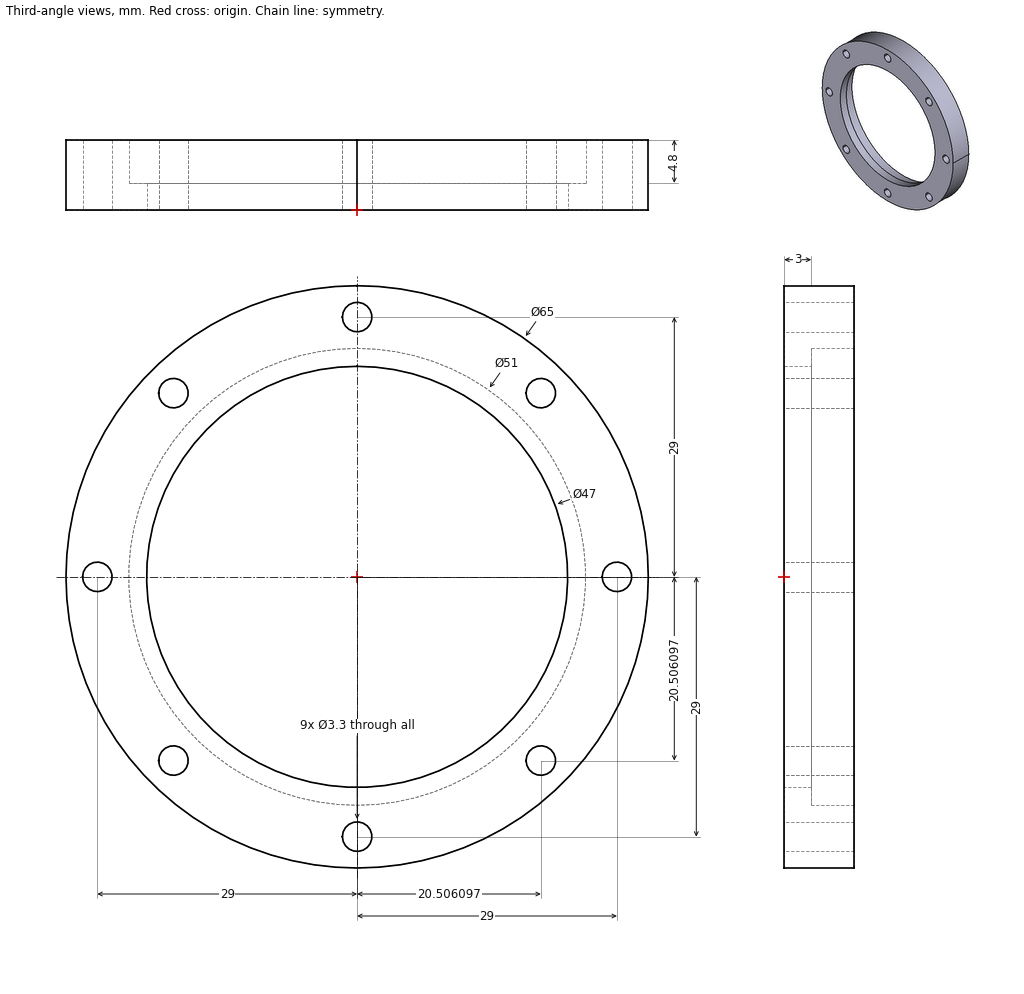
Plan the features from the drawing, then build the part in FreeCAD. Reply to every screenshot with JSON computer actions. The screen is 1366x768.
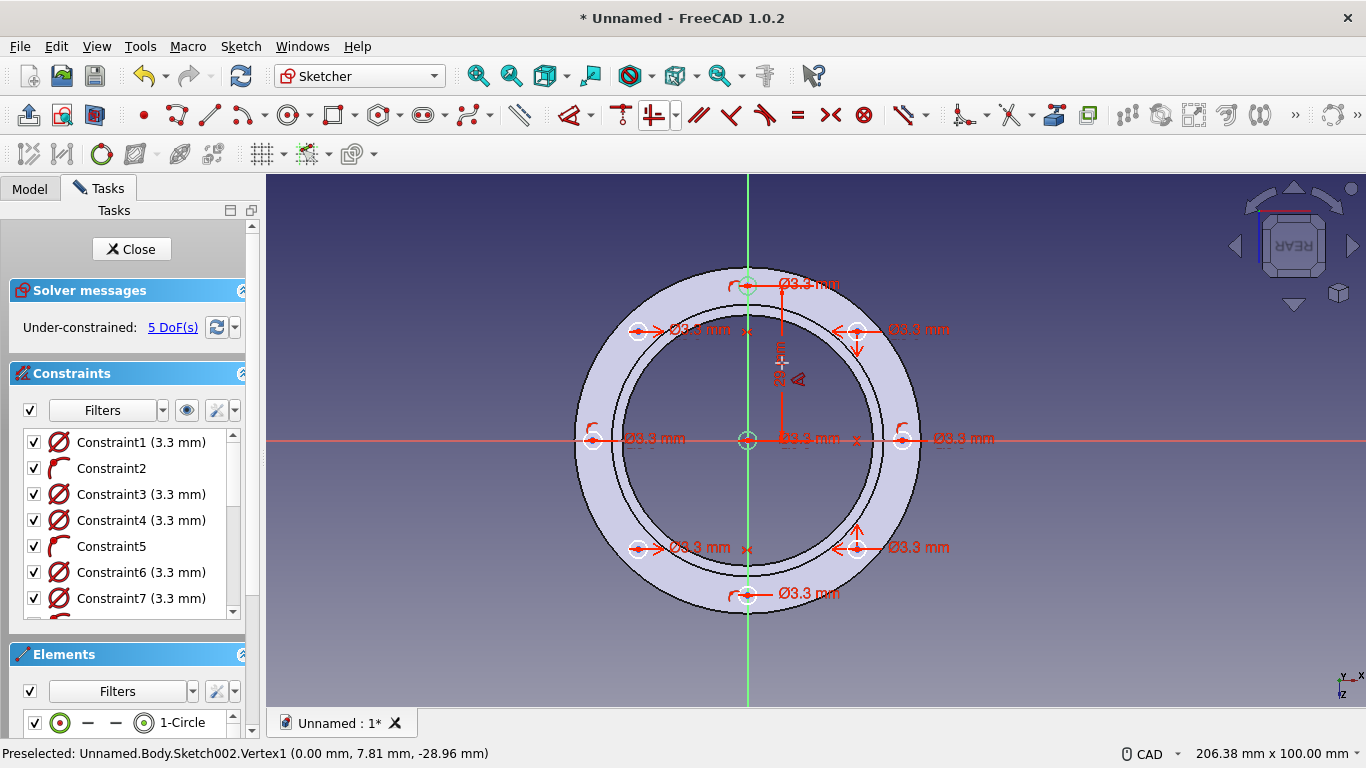
{"action": "left_click", "coordinate": [902, 440]}
{"action": "left_click", "coordinate": [825, 474]}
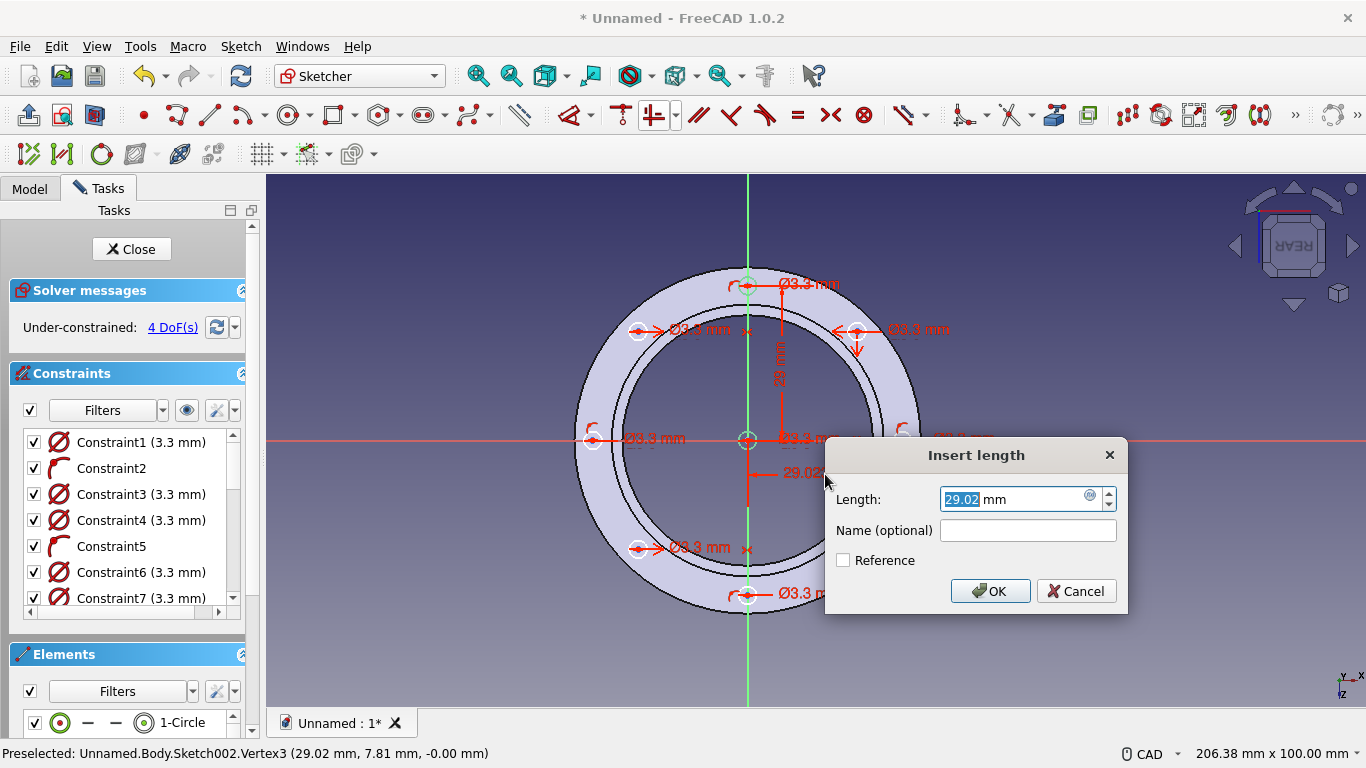
{"action": "type", "text": "29"}
{"action": "key", "text": "Return"}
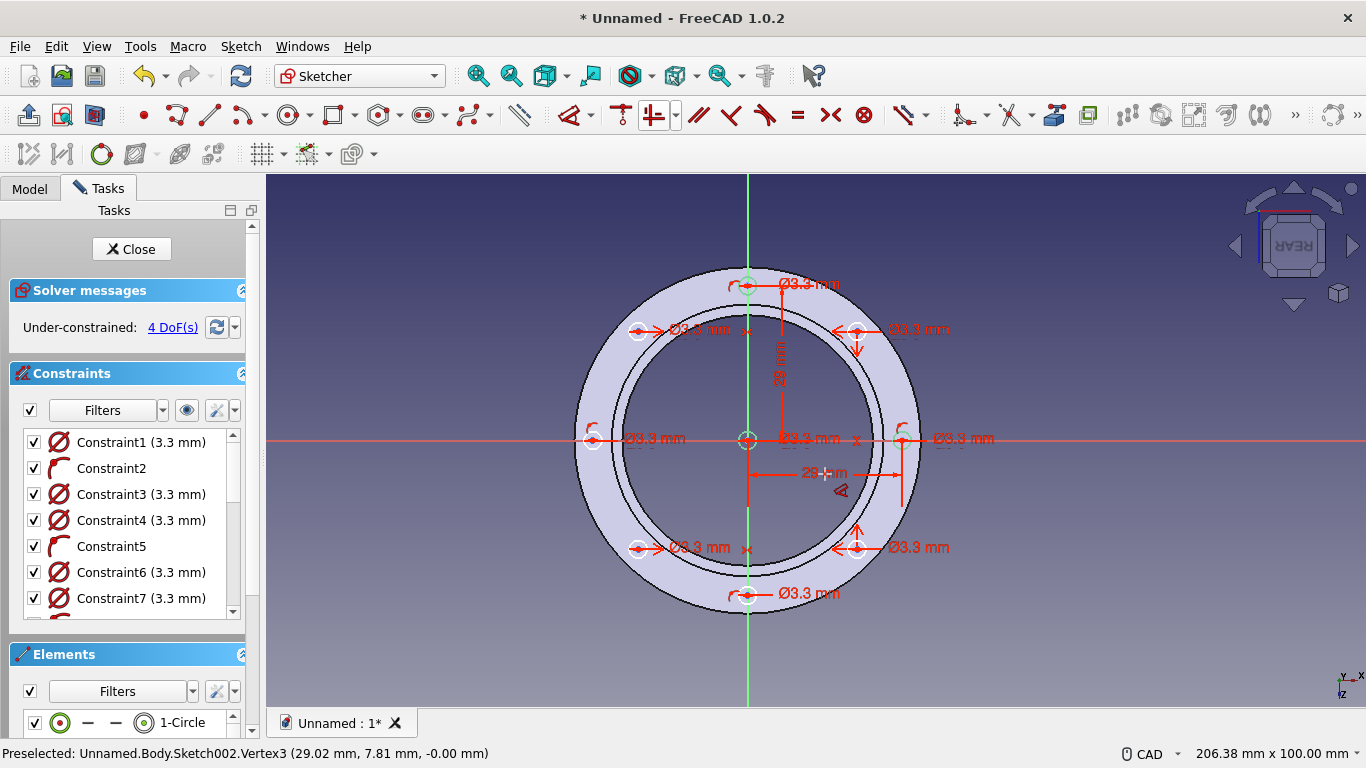
{"action": "left_click", "coordinate": [748, 595]}
{"action": "left_click", "coordinate": [782, 518]}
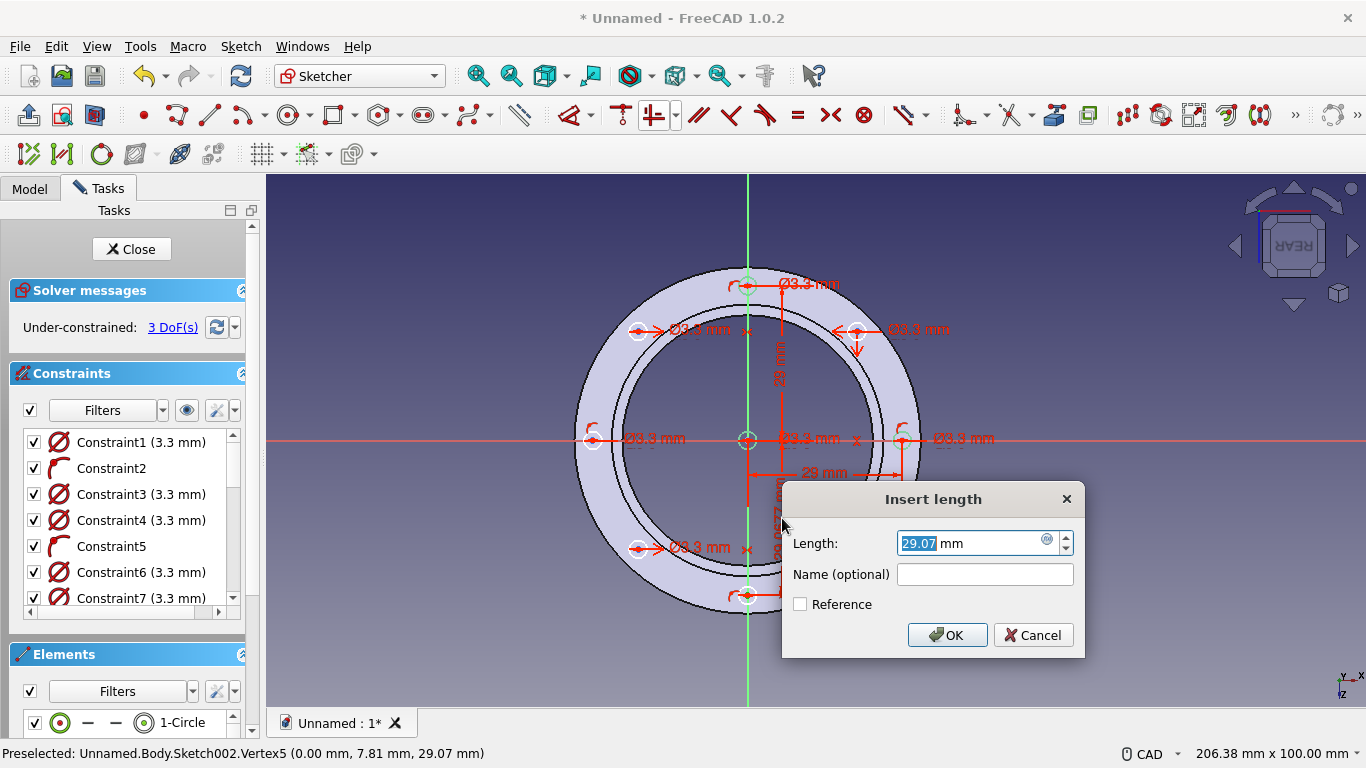
{"action": "type", "text": "29"}
{"action": "key", "text": "Return"}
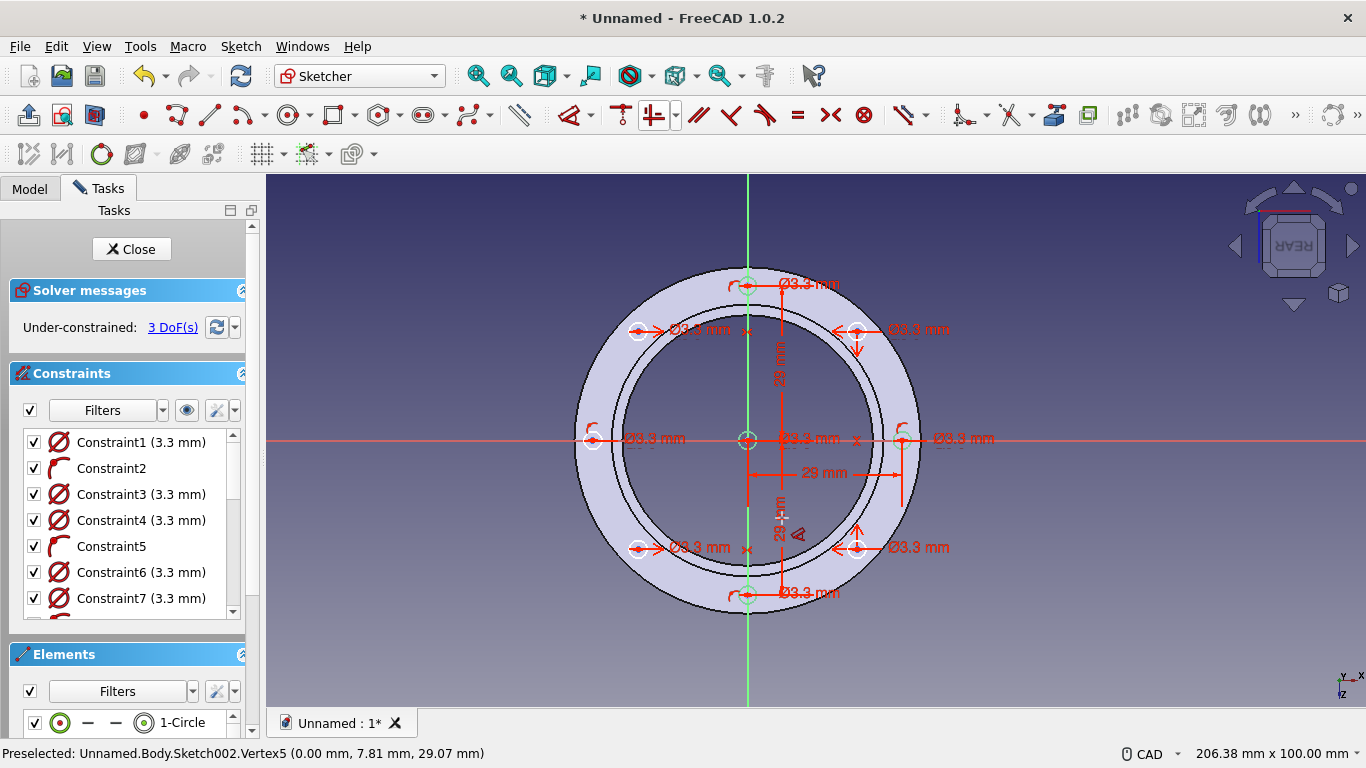
{"action": "left_click", "coordinate": [593, 440]}
{"action": "left_click", "coordinate": [670, 474]}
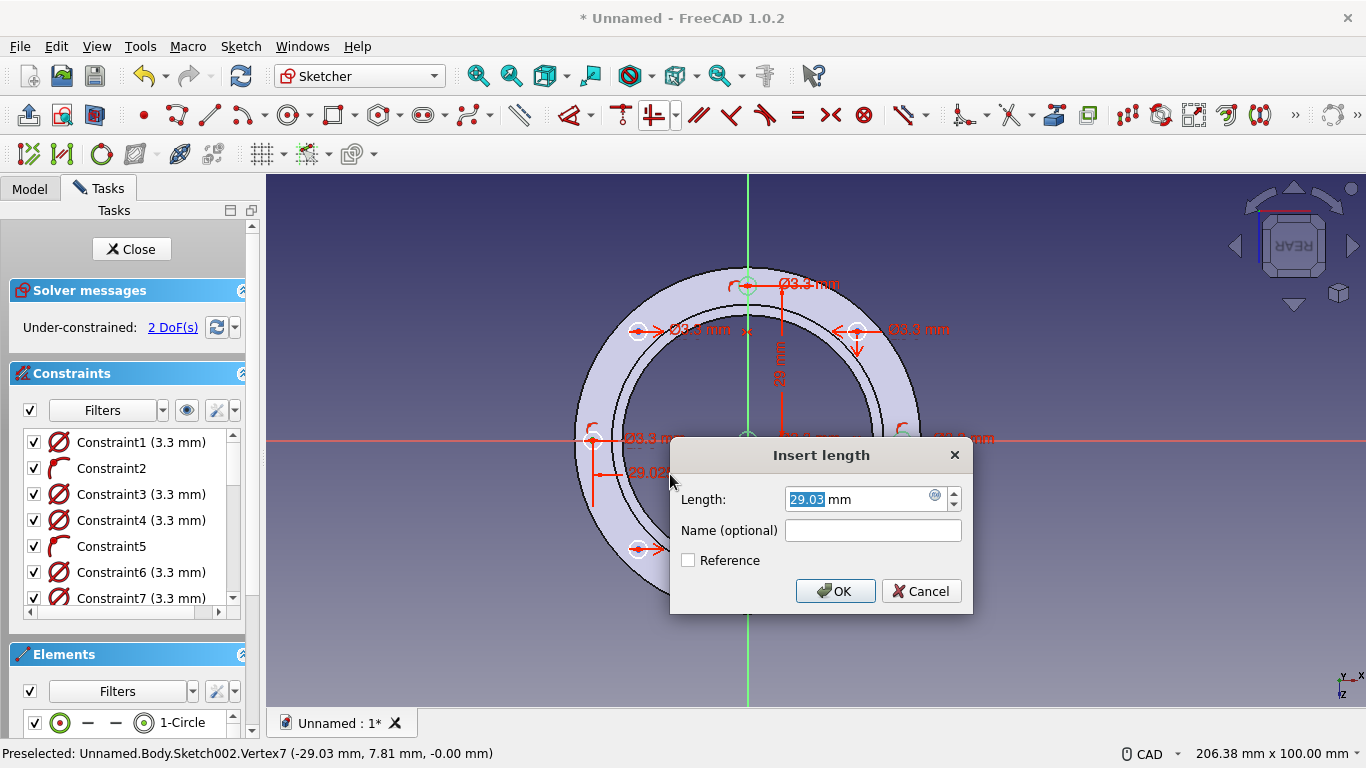
{"action": "type", "text": "29"}
{"action": "key", "text": "Return"}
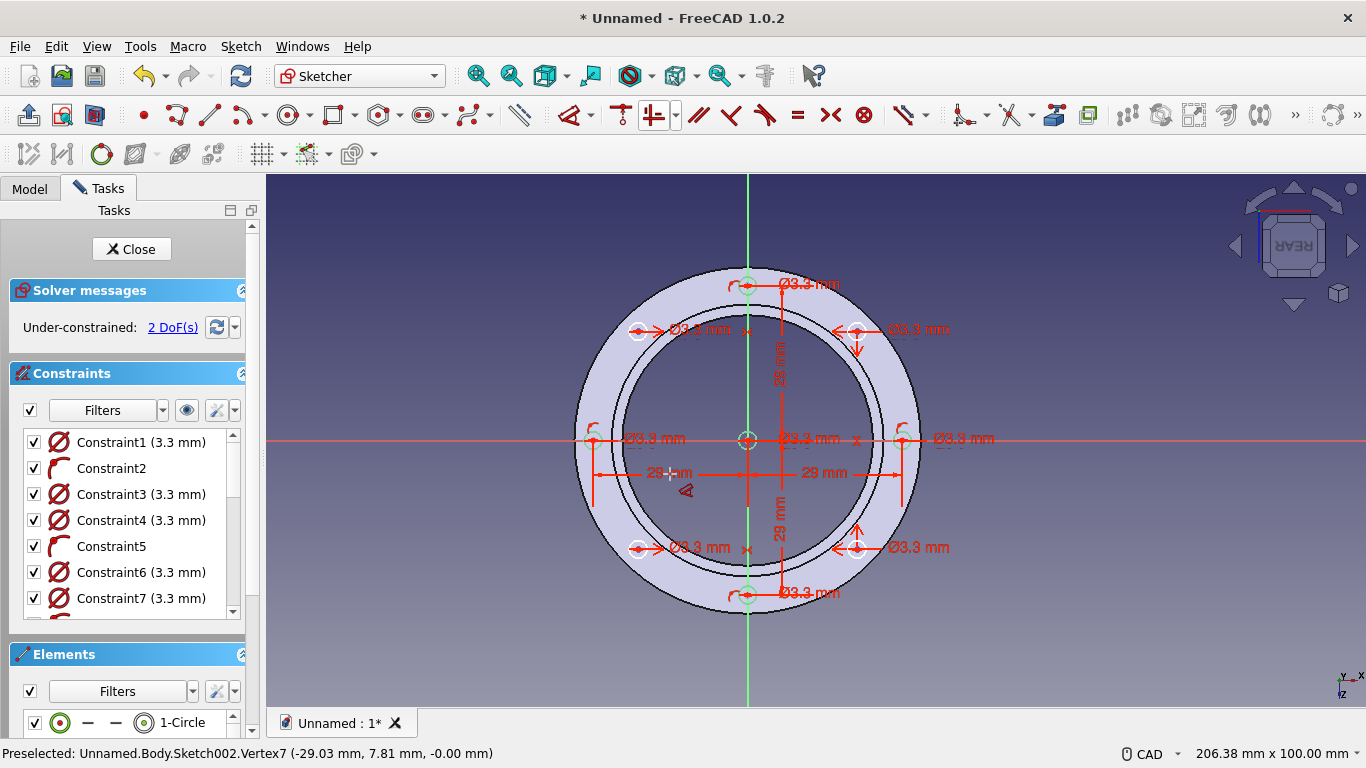
{"action": "left_click", "coordinate": [857, 332]}
{"action": "left_click", "coordinate": [802, 298]}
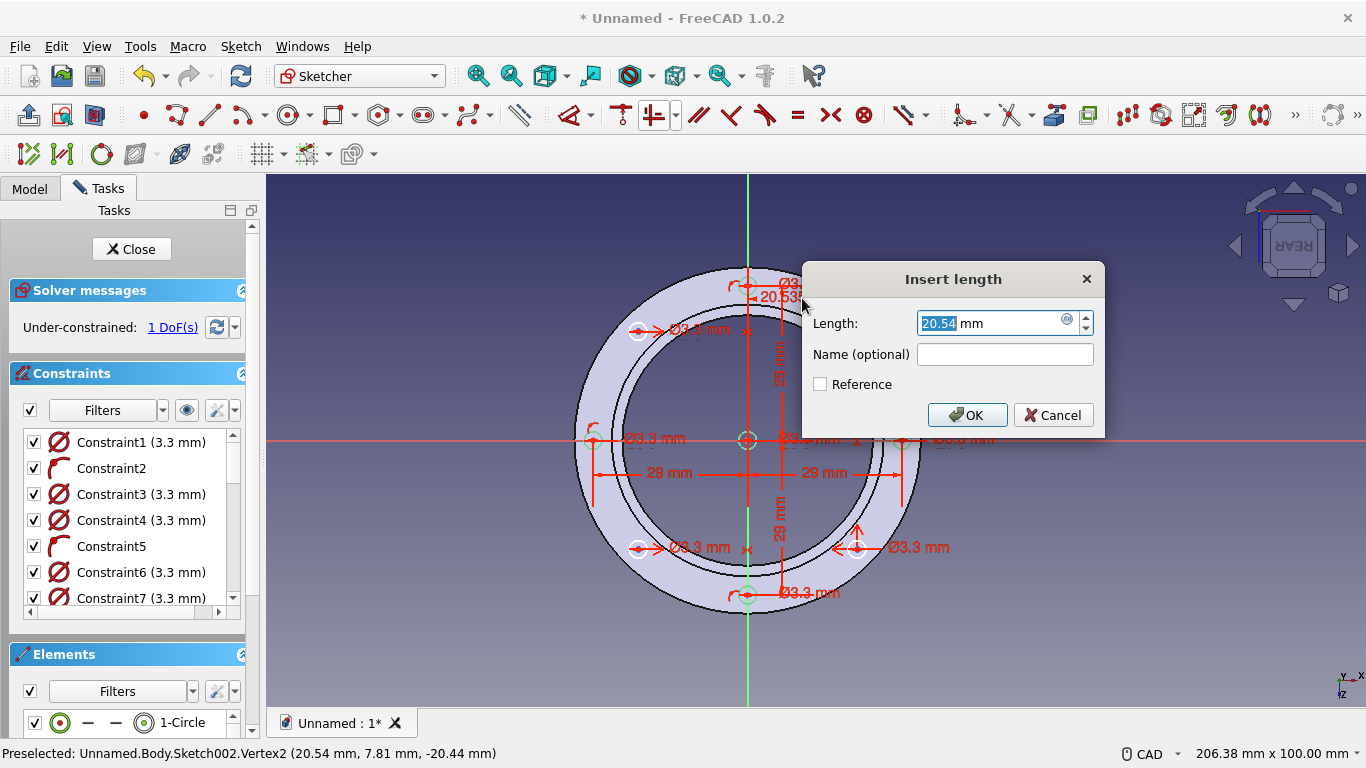
{"action": "type", "text": "20.506097"}
{"action": "key", "text": "Return"}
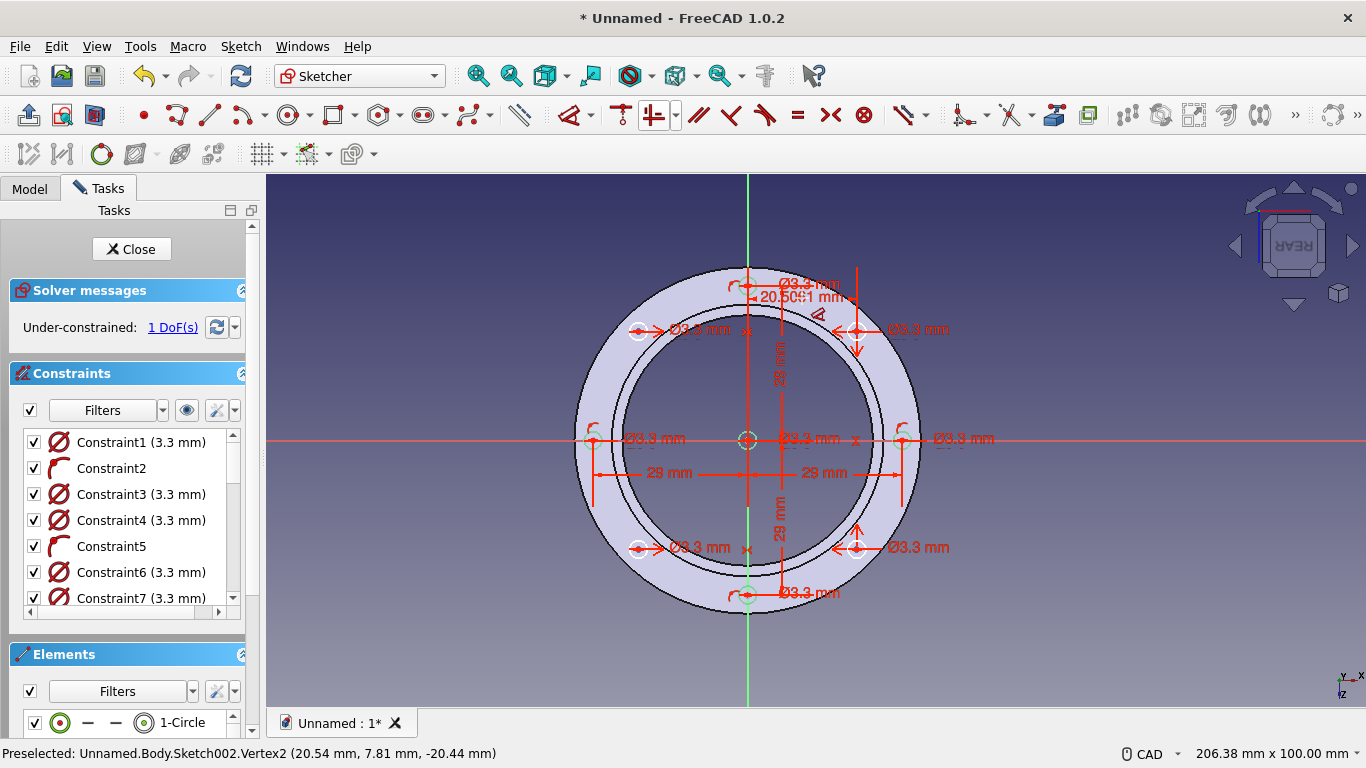
{"action": "left_click", "coordinate": [857, 332]}
{"action": "left_click", "coordinate": [891, 386]}